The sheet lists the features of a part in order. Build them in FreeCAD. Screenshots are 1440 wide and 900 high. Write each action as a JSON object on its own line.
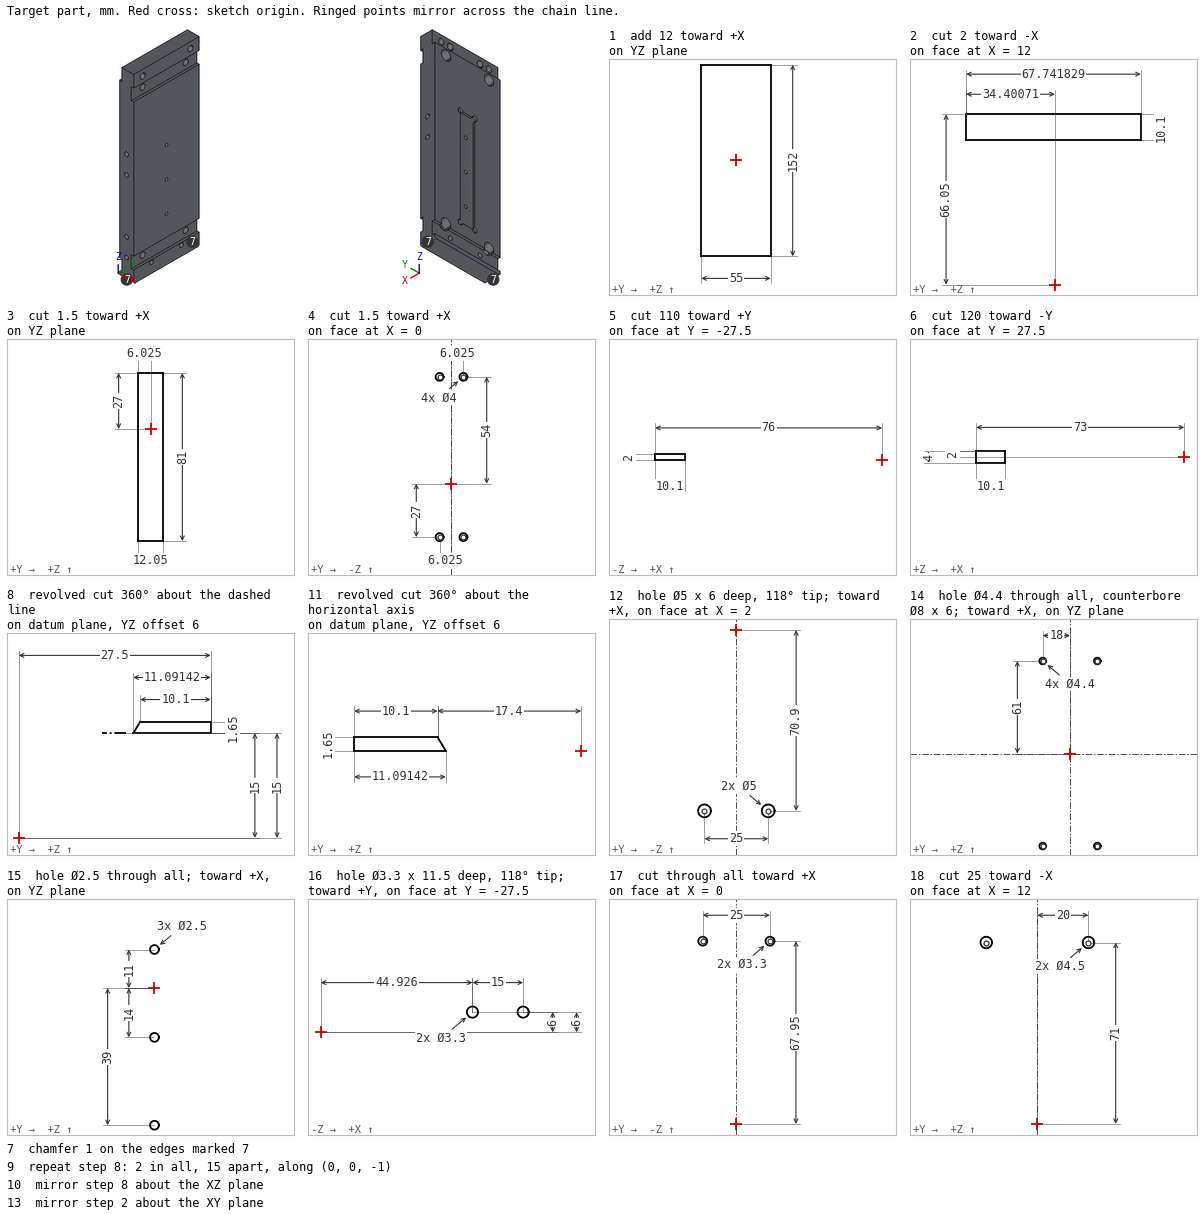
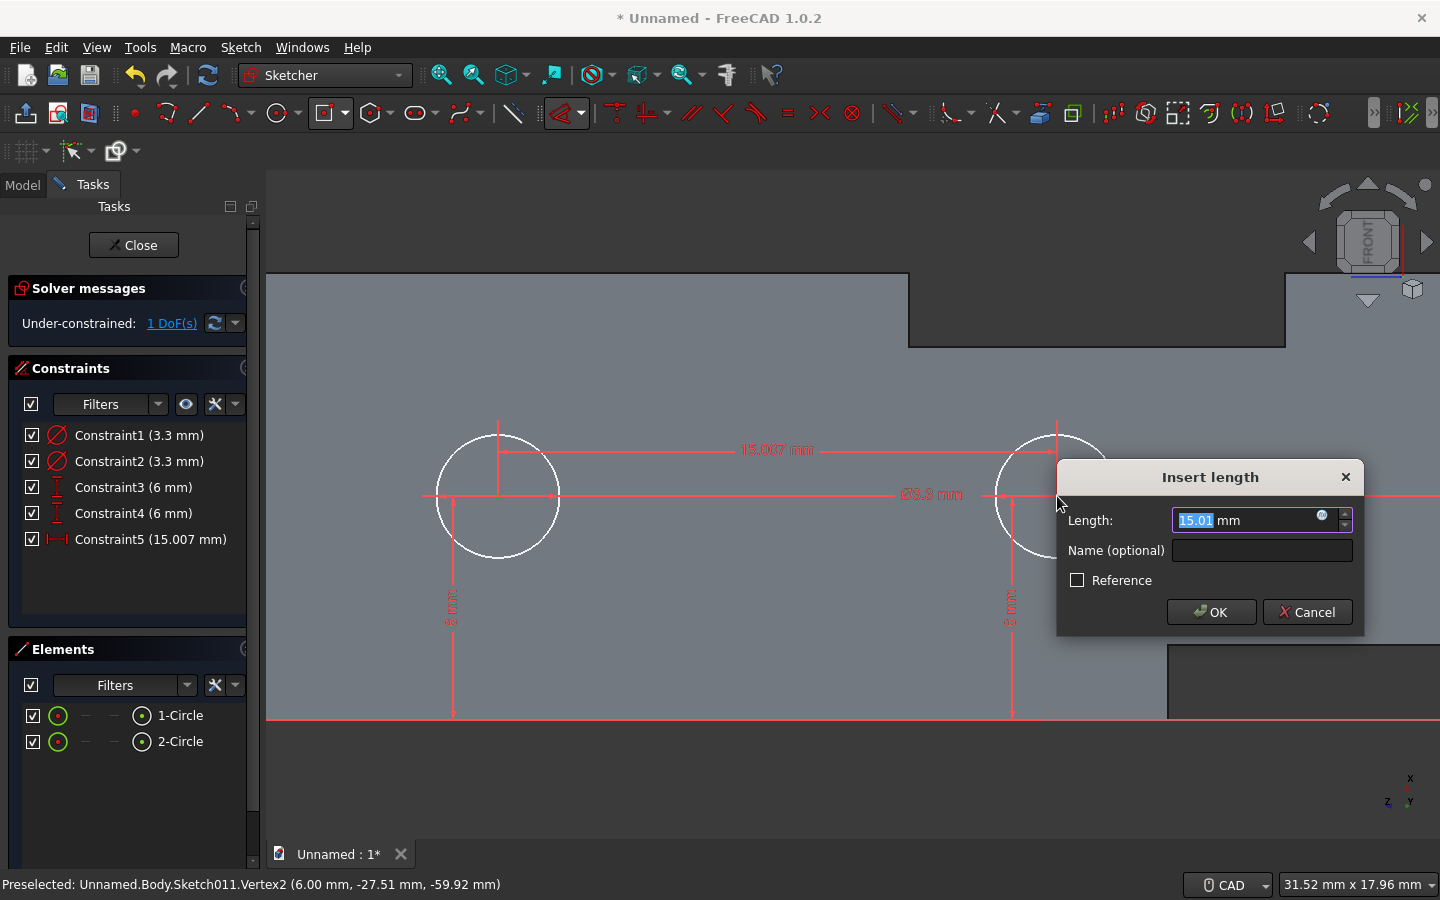
{"action": "type", "text": "15"}
{"action": "key", "text": "Return"}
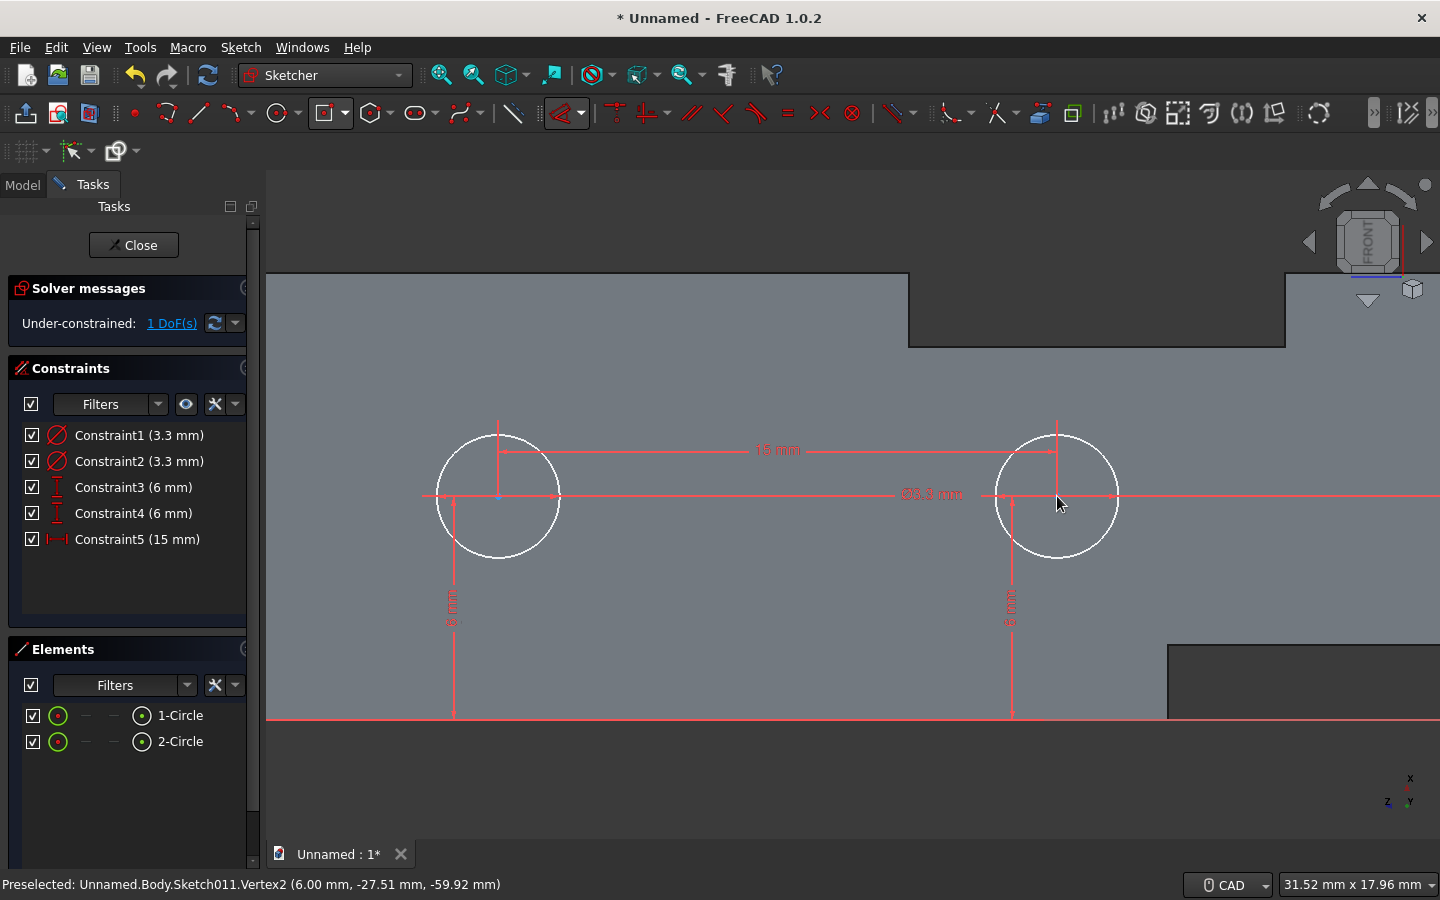
{"action": "left_click", "coordinate": [498, 496]}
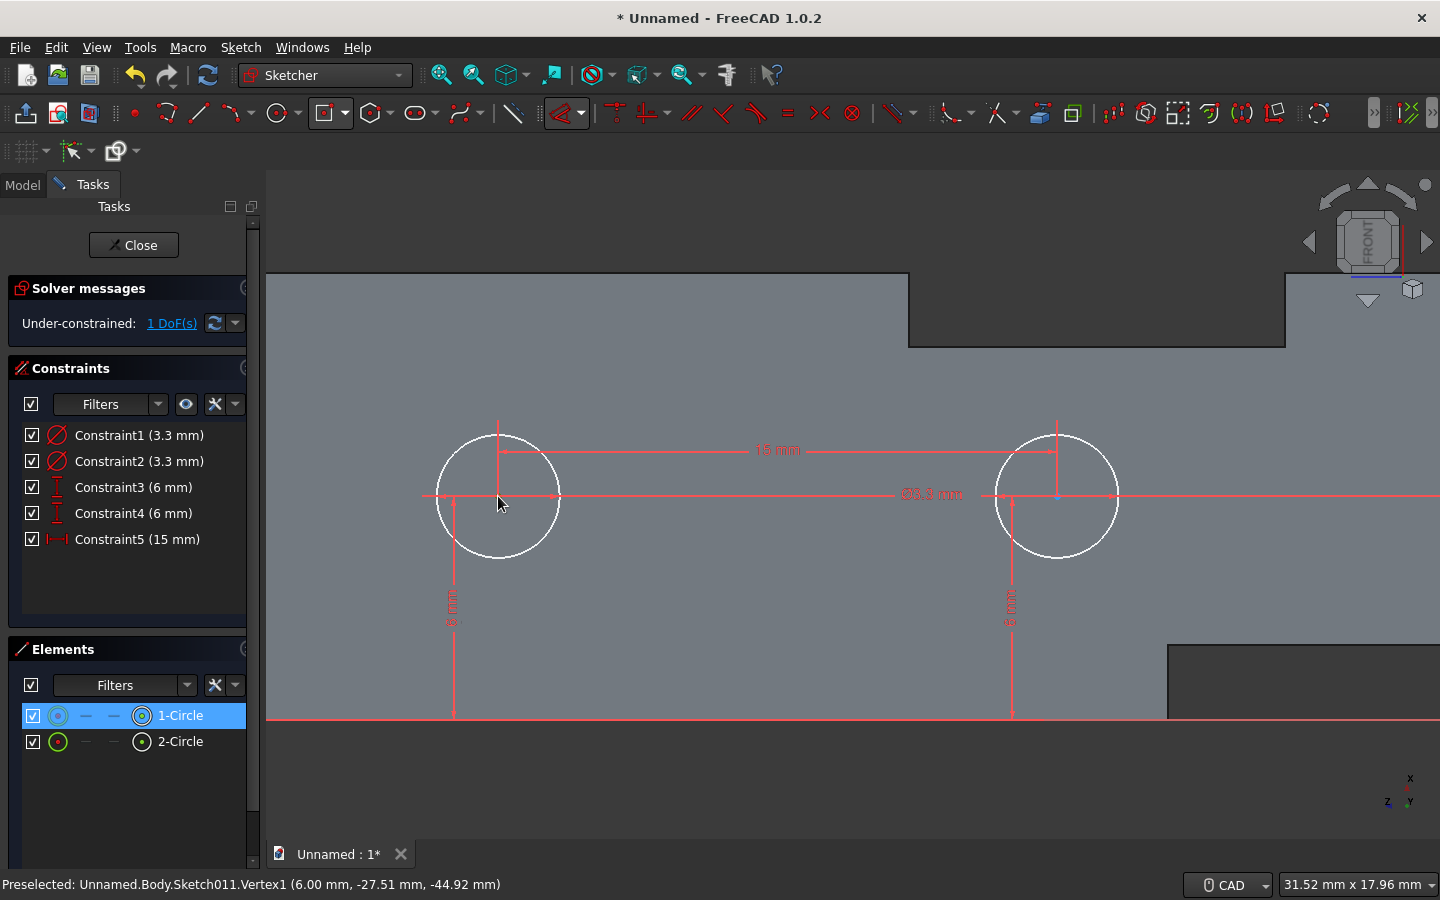
{"action": "key", "text": "l"}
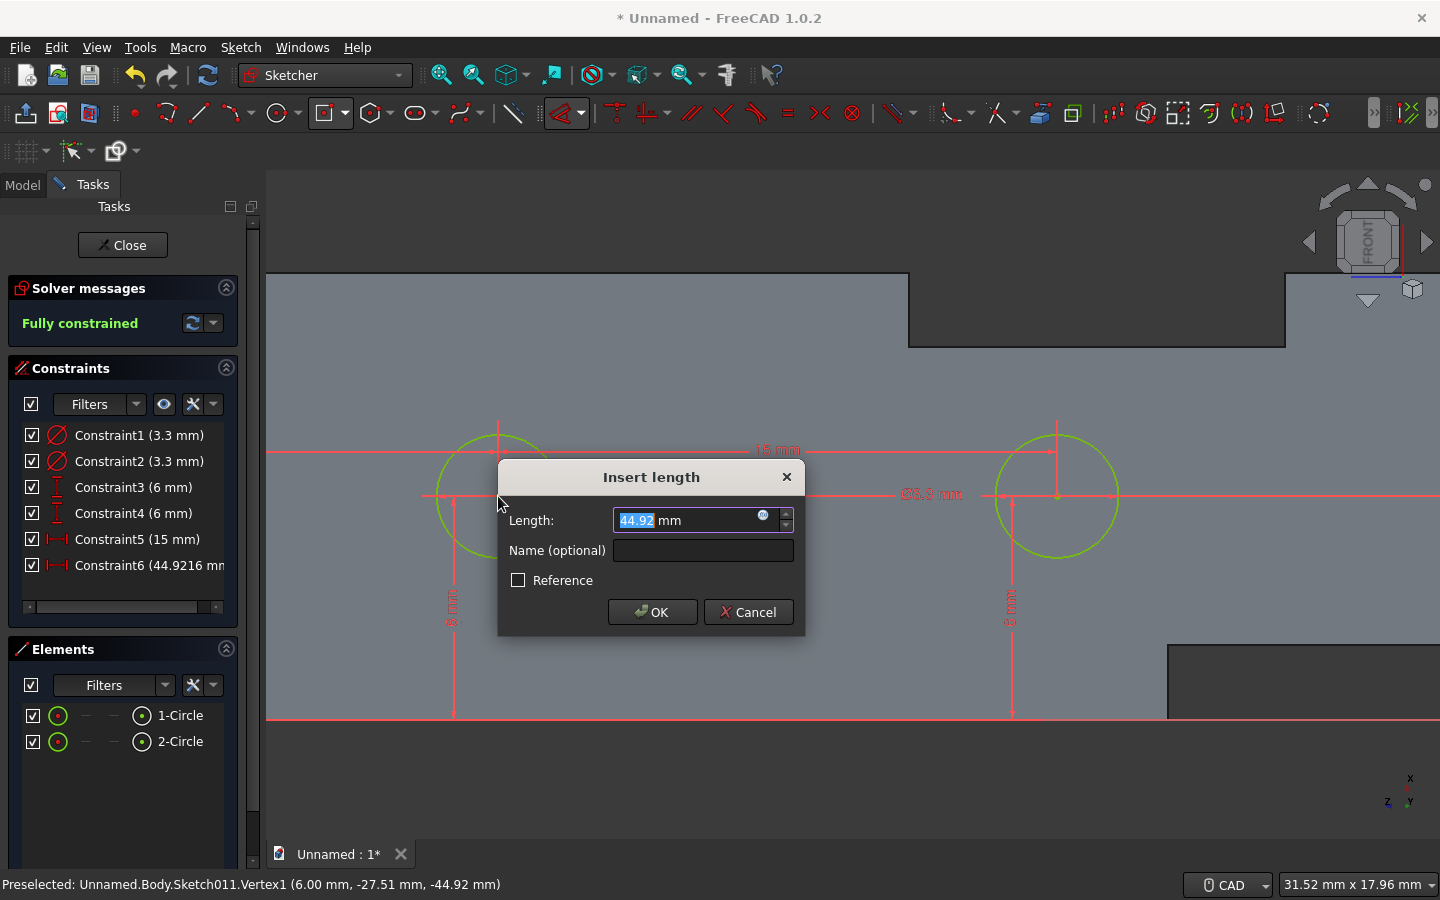
{"action": "type", "text": "44.926"}
{"action": "key", "text": "Return"}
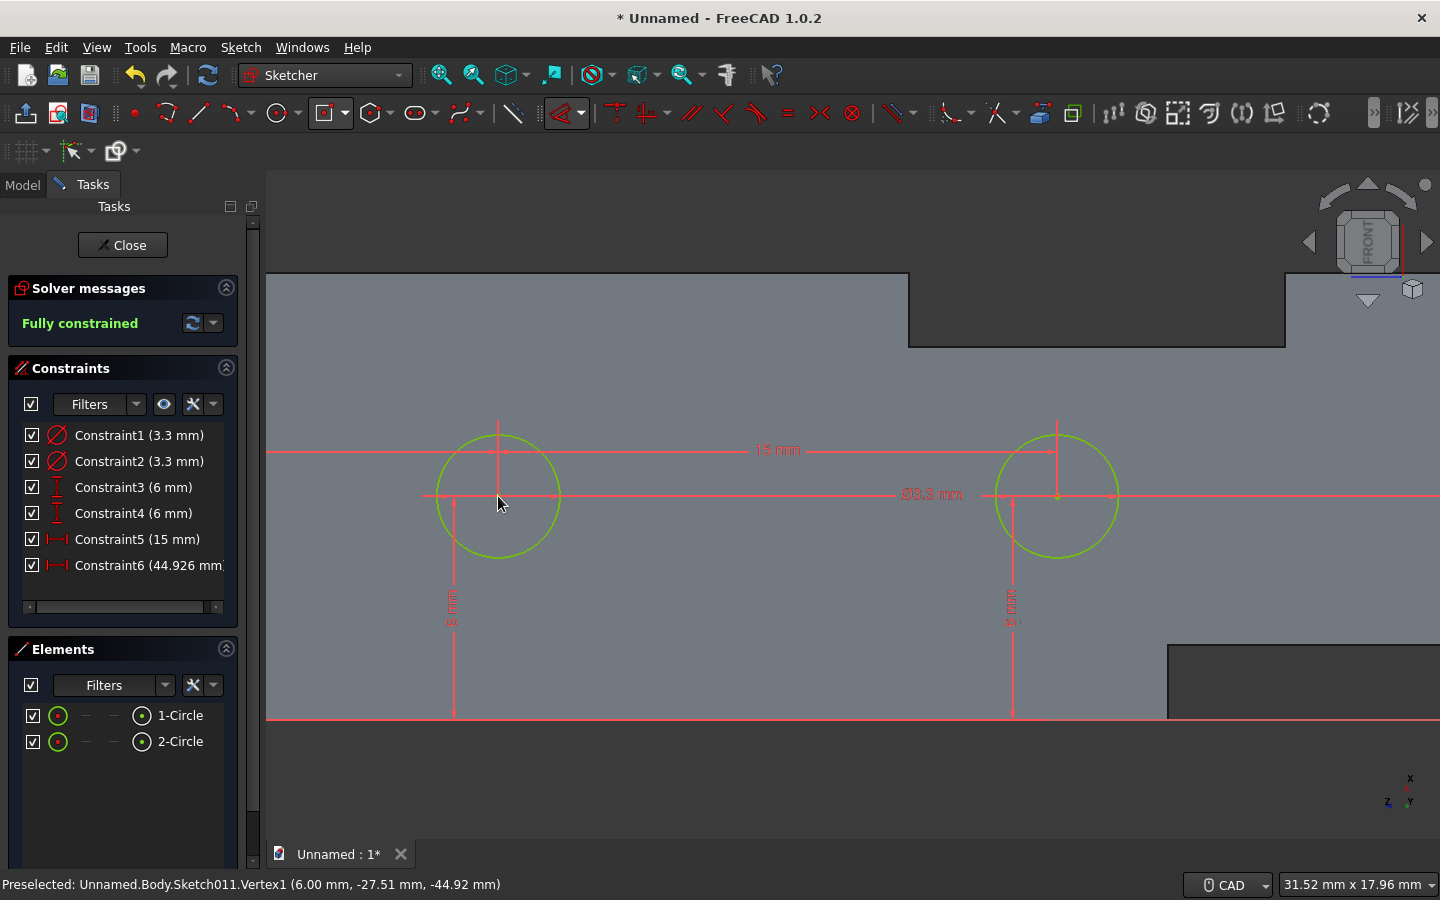
{"action": "left_click", "coordinate": [123, 245]}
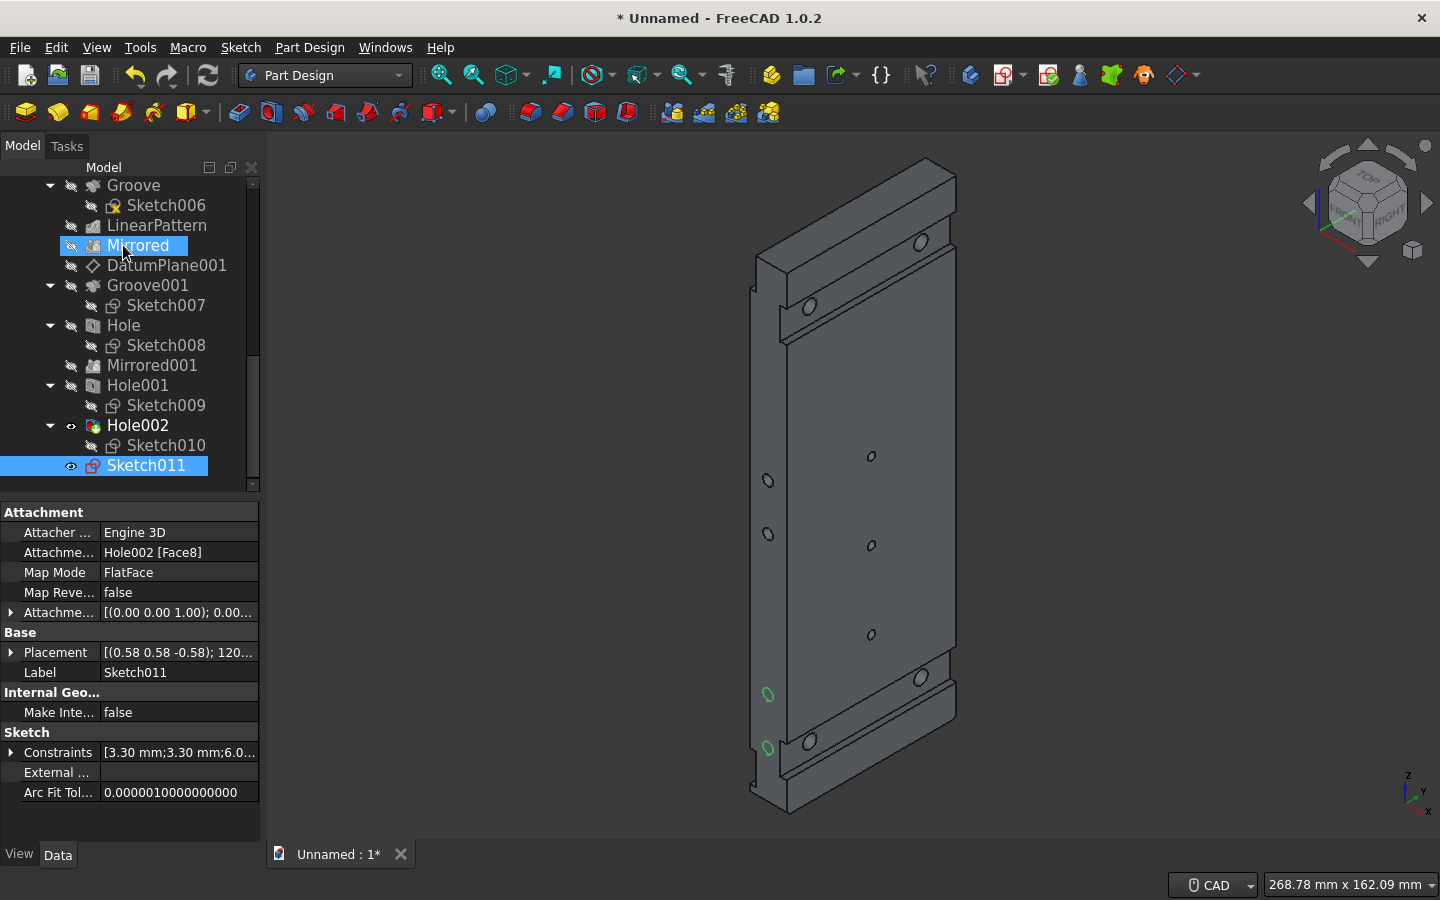
{"action": "left_click", "coordinate": [272, 112]}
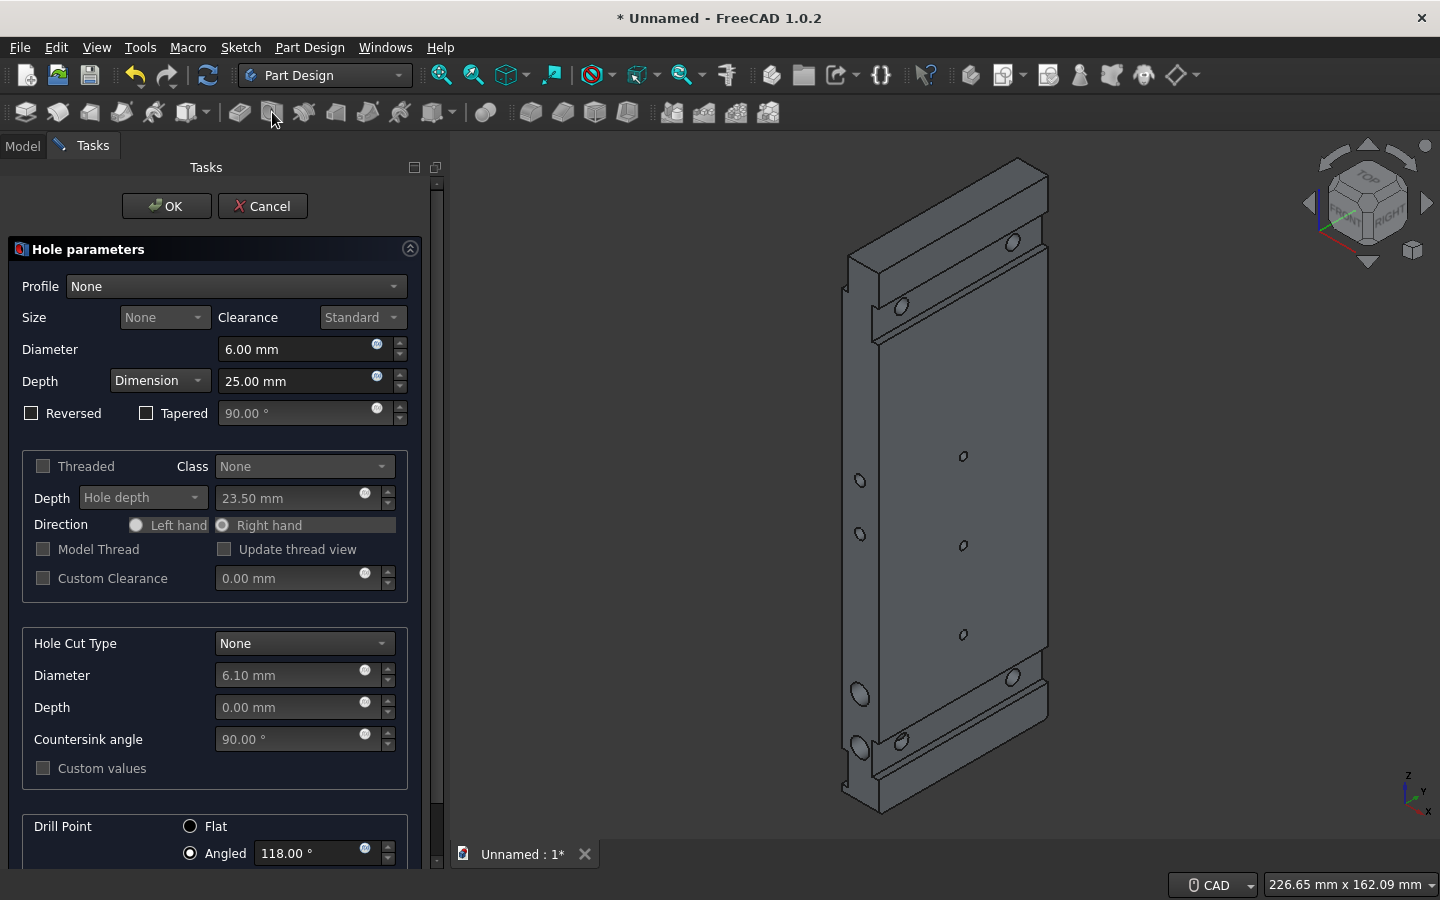
{"action": "triple_click", "coordinate": [305, 349]}